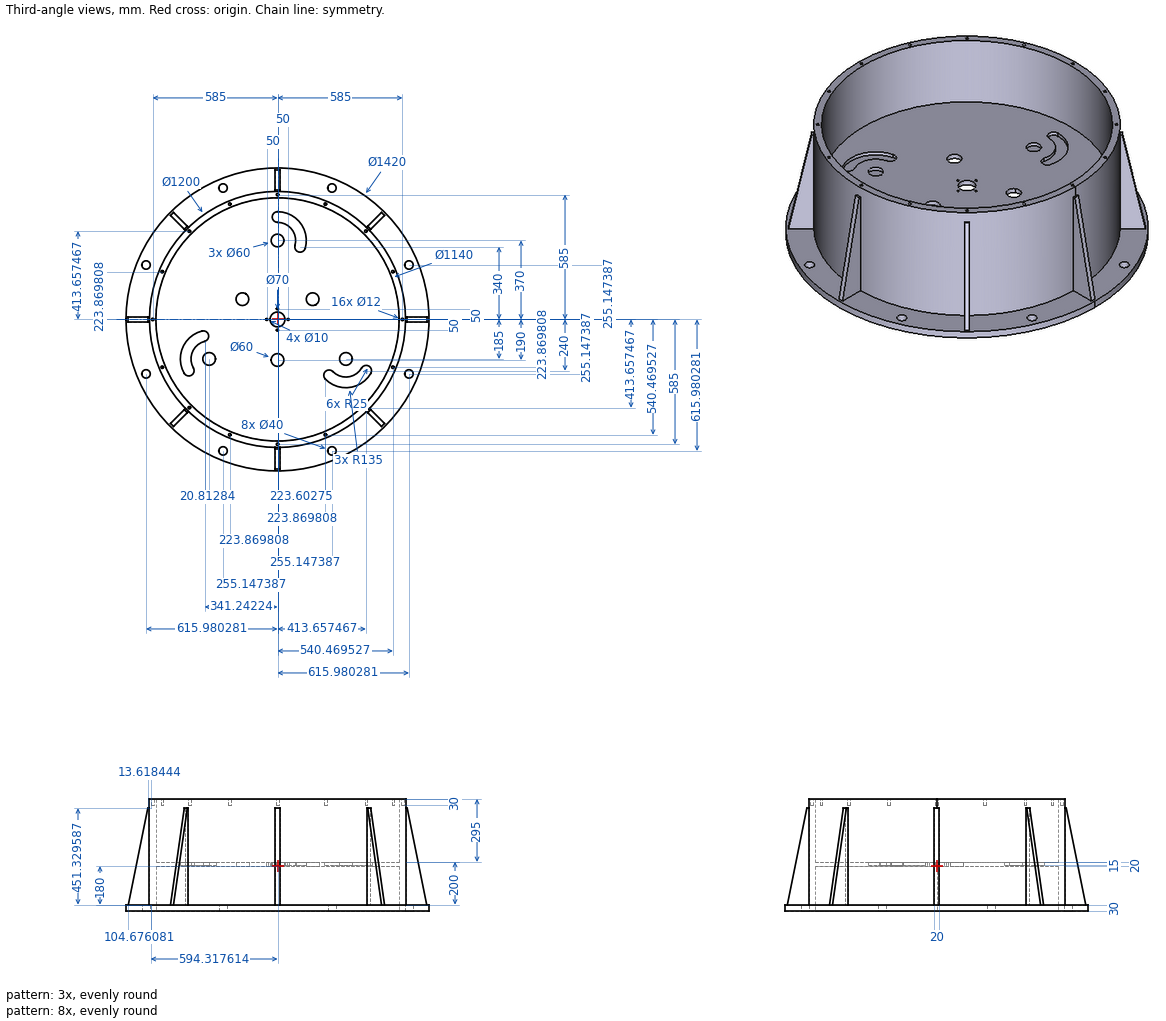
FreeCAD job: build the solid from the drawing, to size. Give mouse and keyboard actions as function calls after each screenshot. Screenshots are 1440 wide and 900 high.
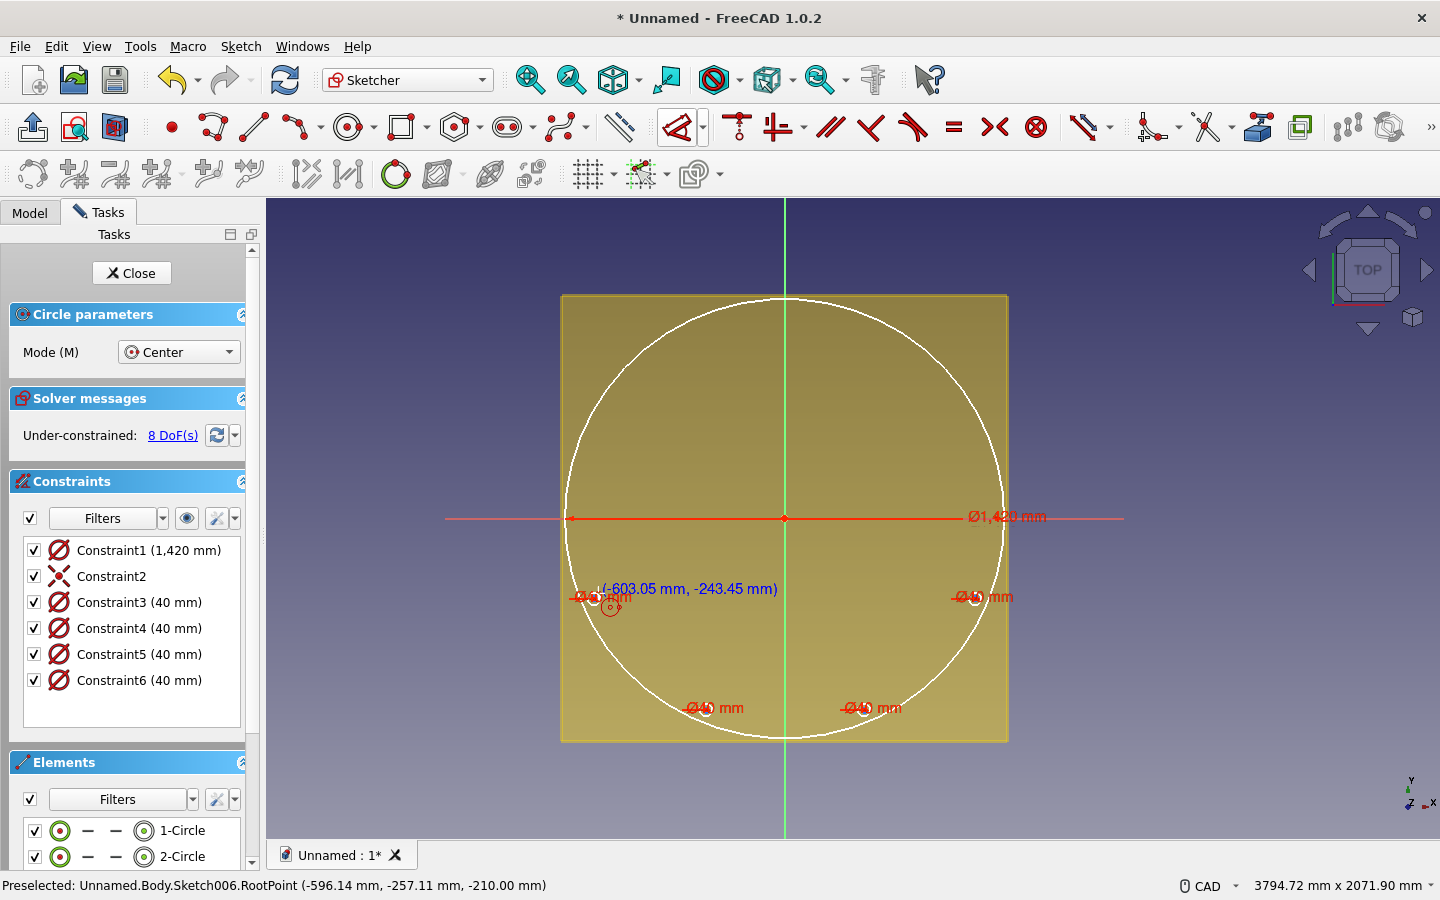
scroll(975, 440, up, 7)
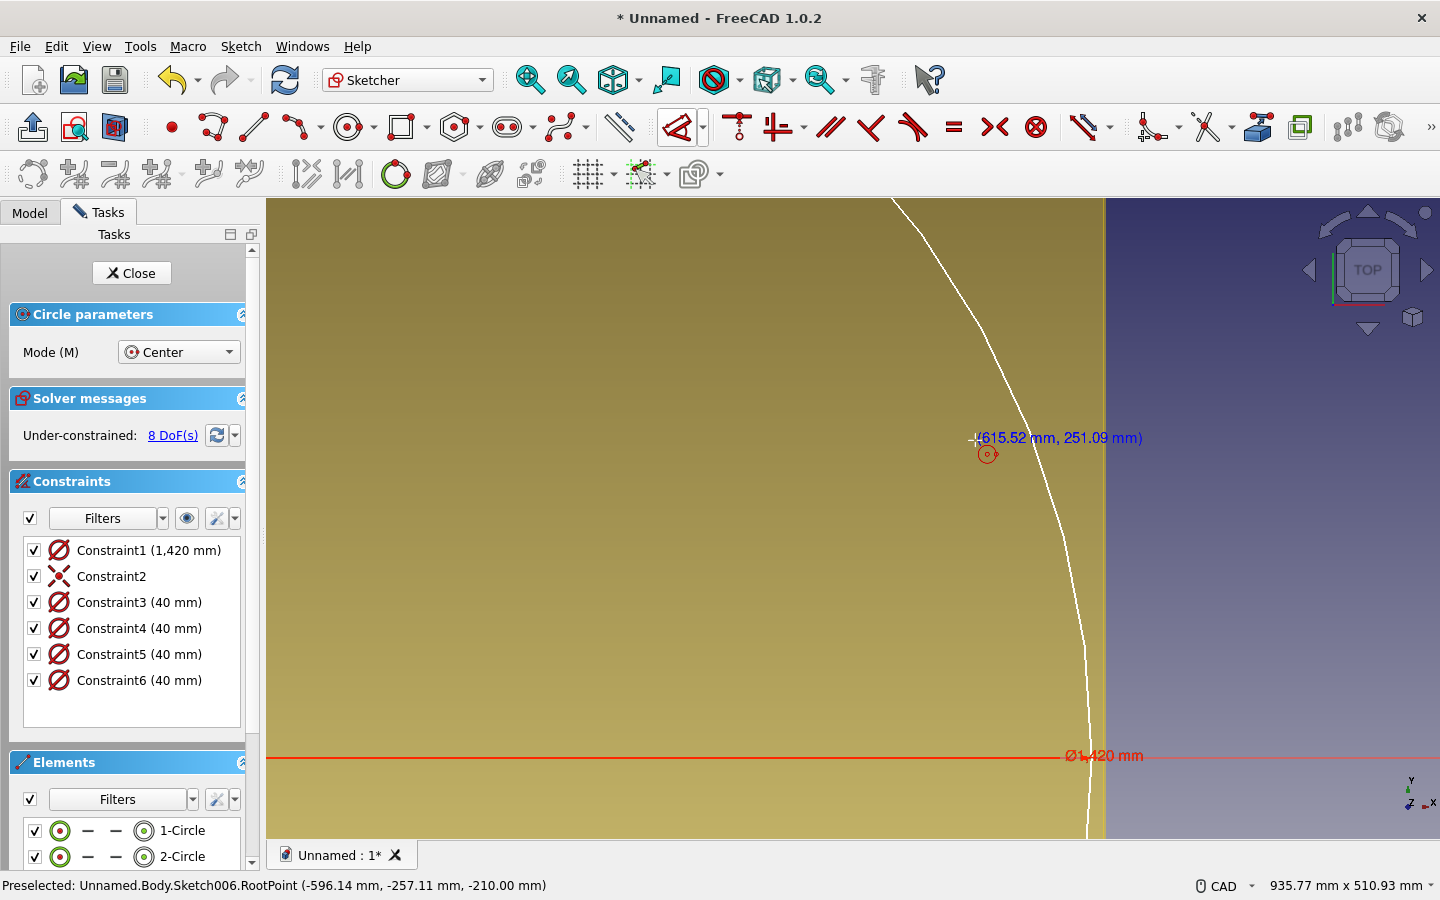
scroll(976, 440, down, 7)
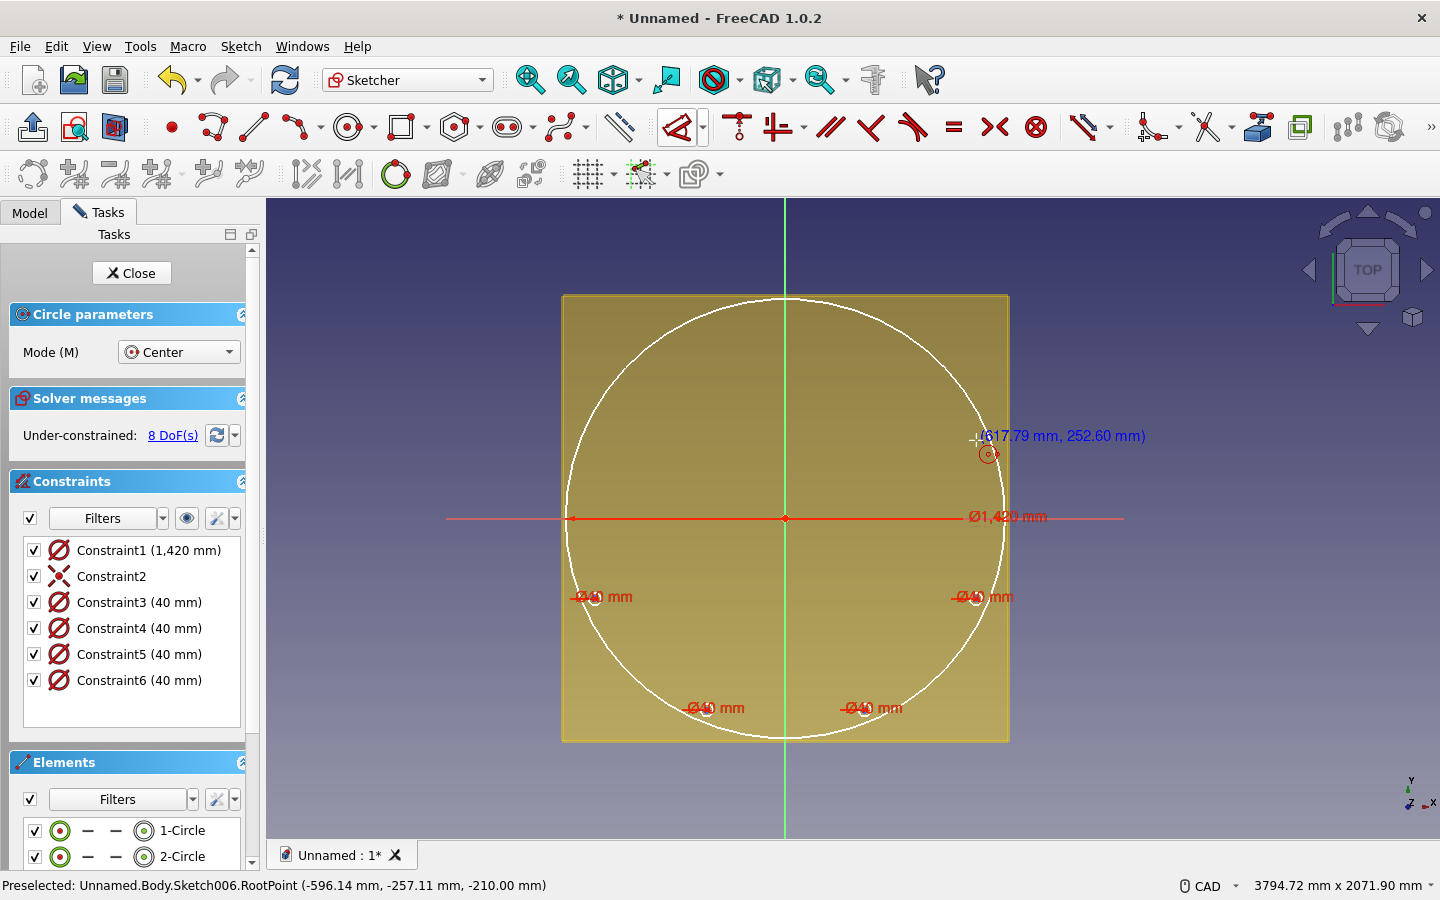
click(976, 440)
move(972, 435)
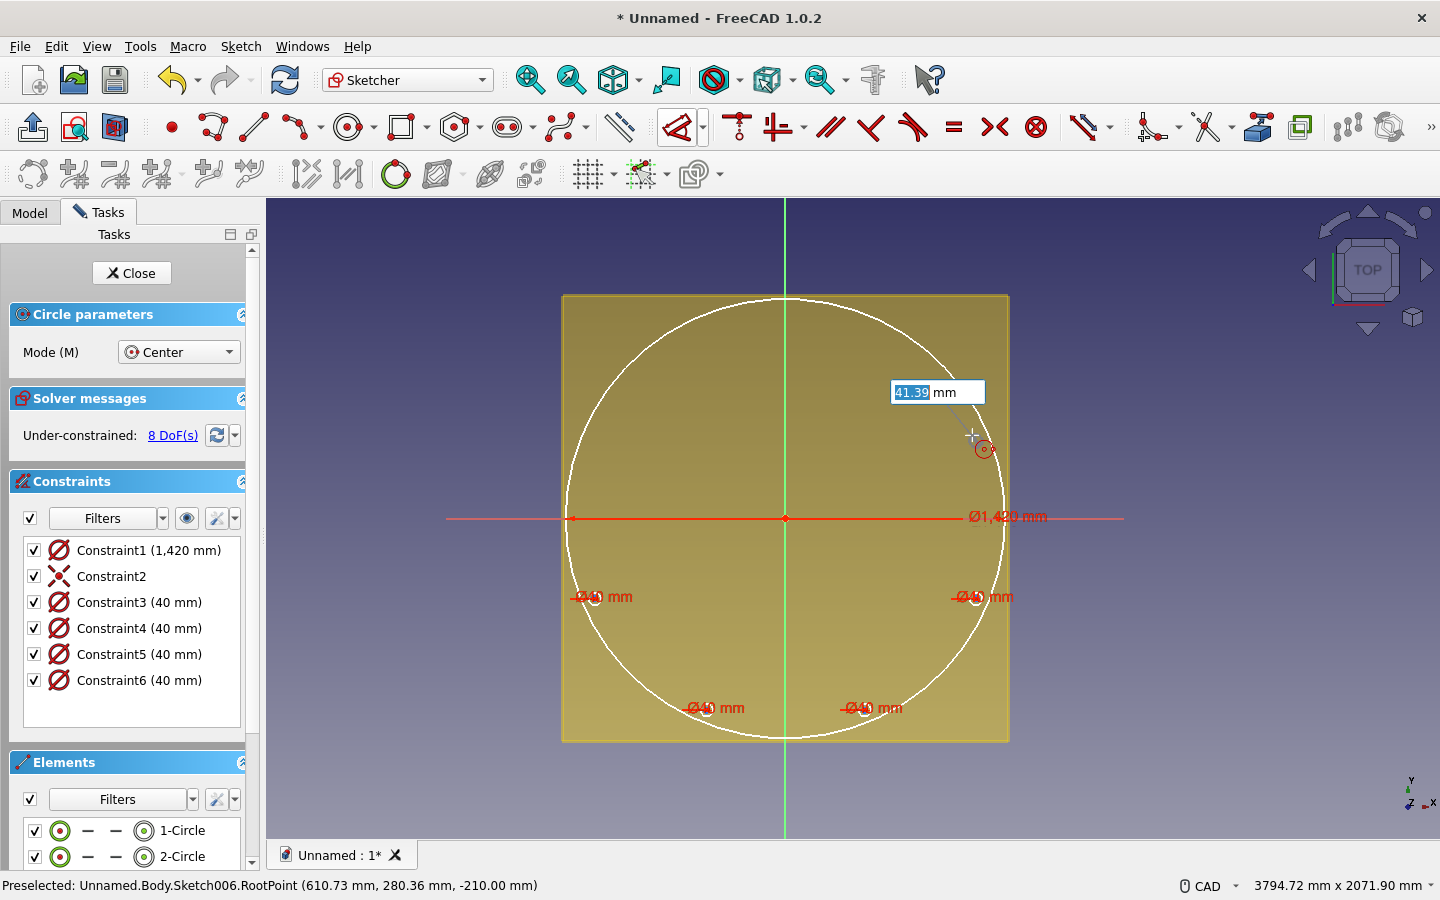
text(40)
key(Return)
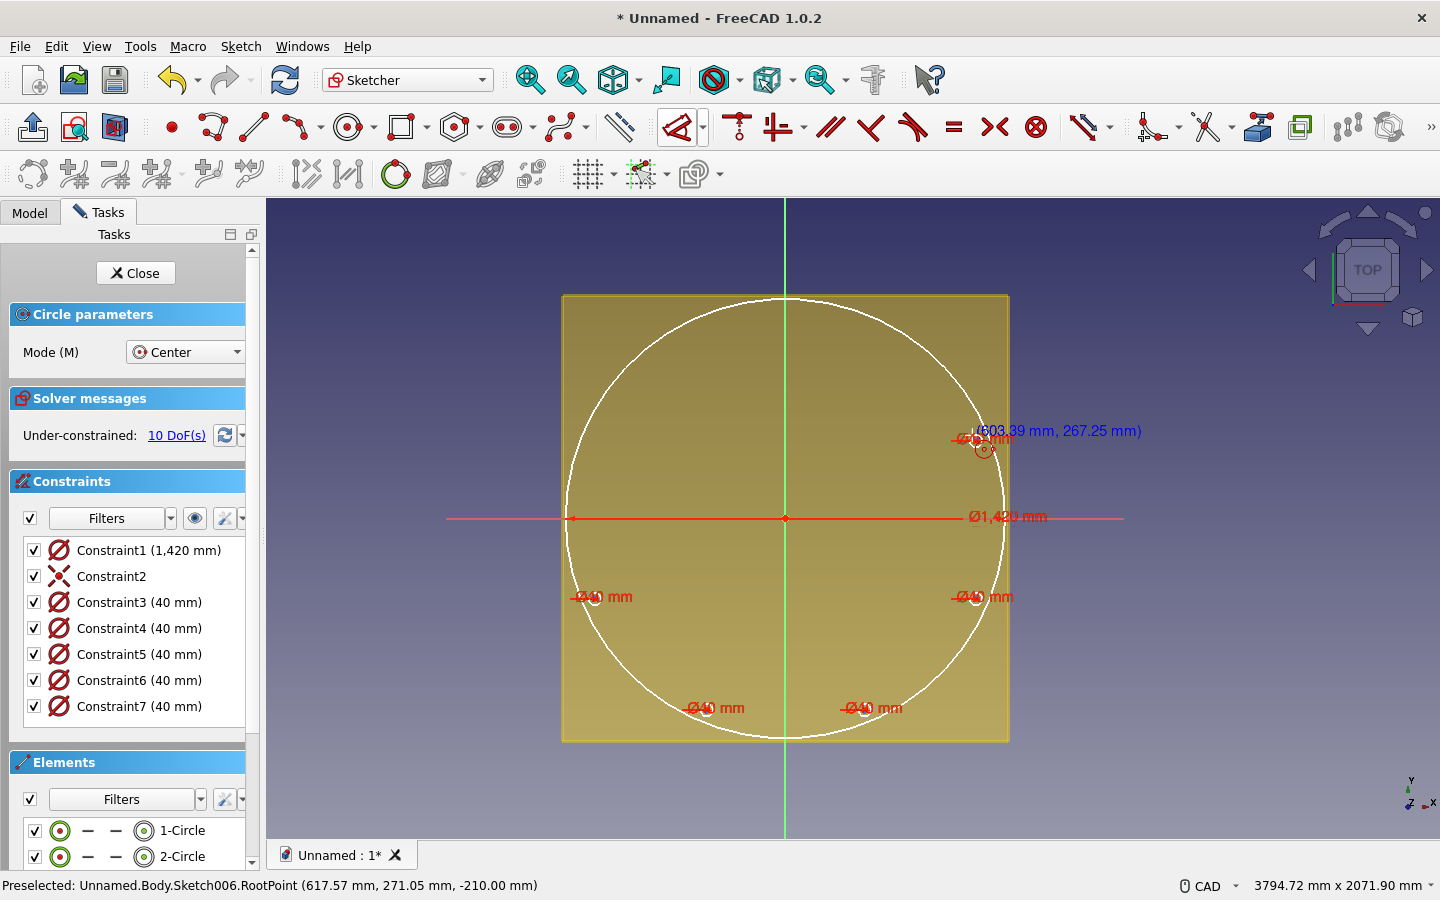
scroll(864, 328, up, 7)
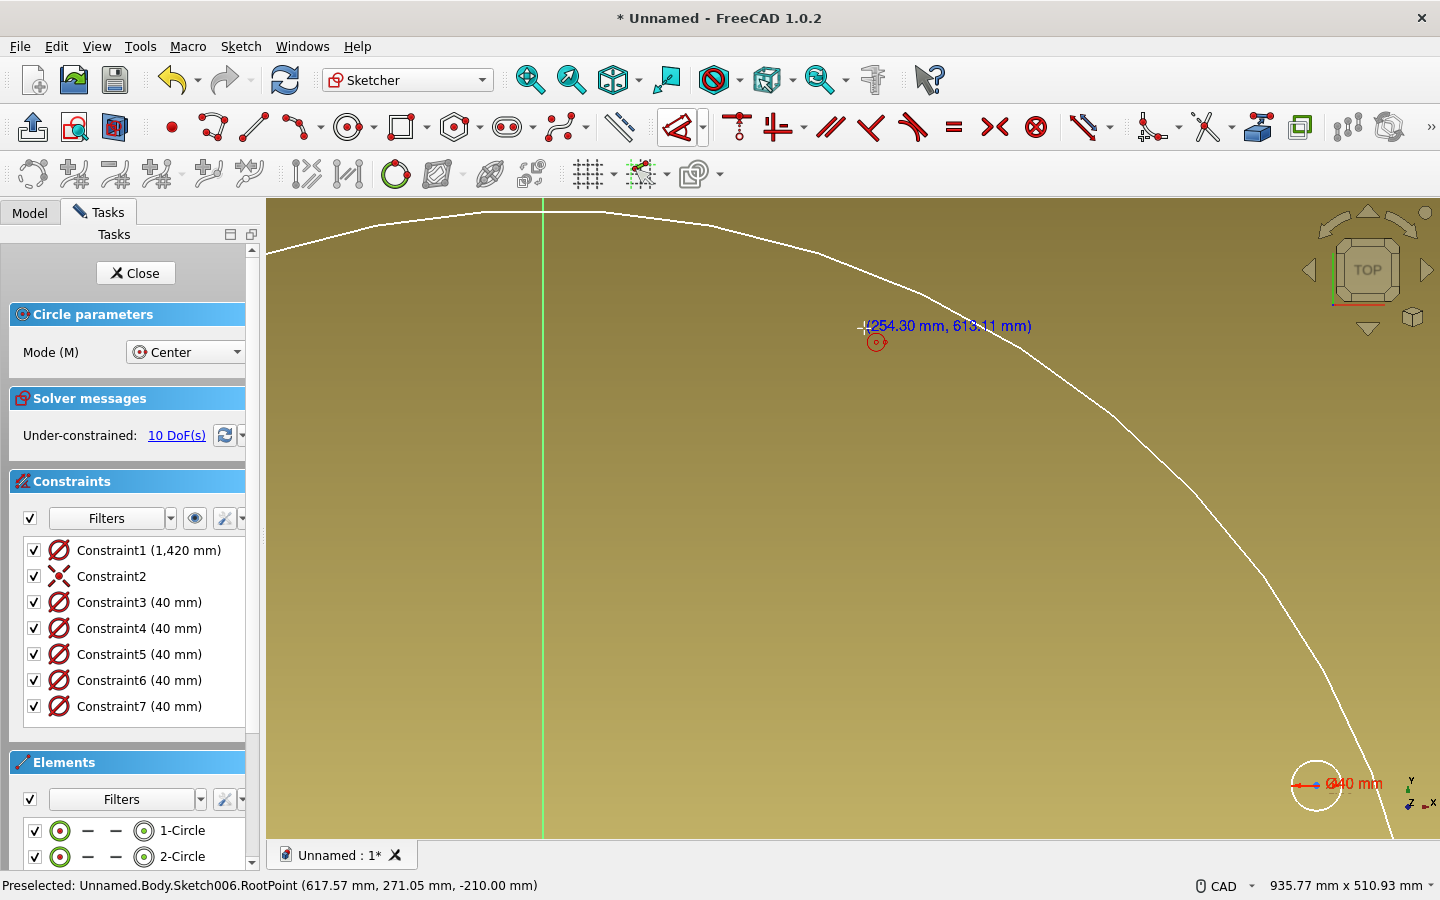
scroll(863, 328, down, 7)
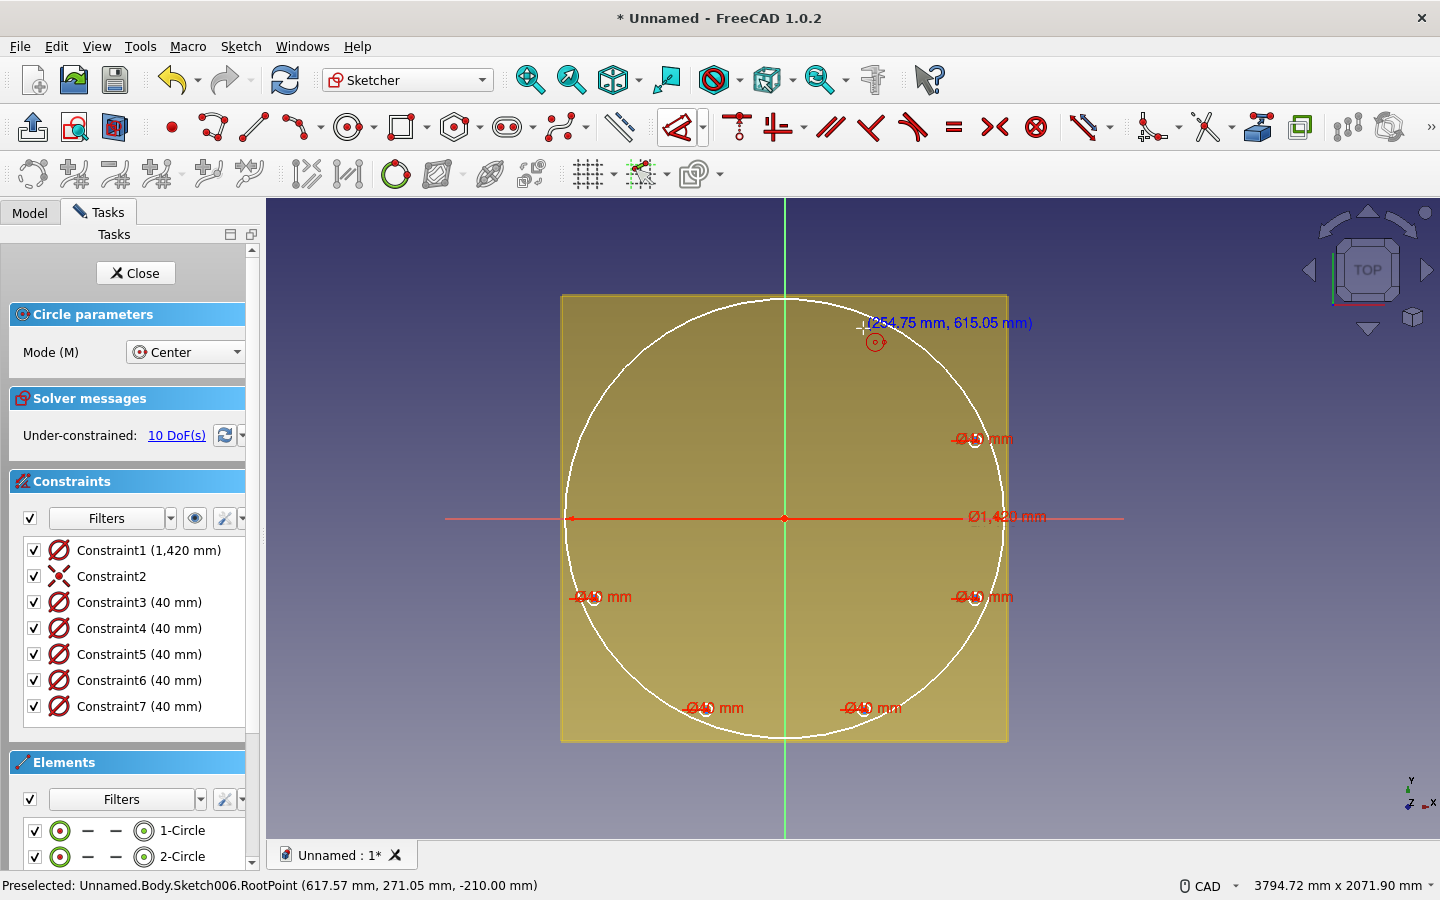
click(864, 328)
move(868, 332)